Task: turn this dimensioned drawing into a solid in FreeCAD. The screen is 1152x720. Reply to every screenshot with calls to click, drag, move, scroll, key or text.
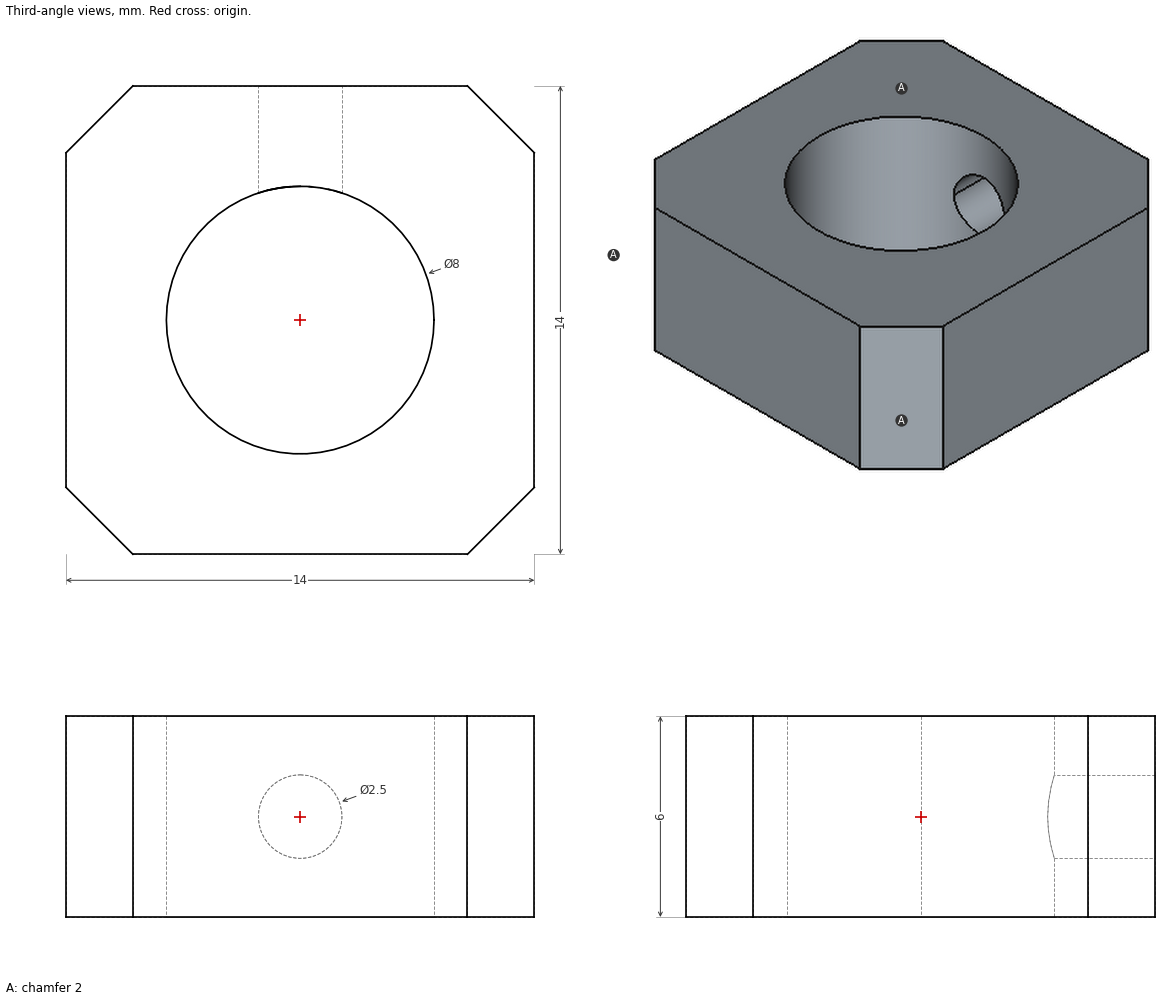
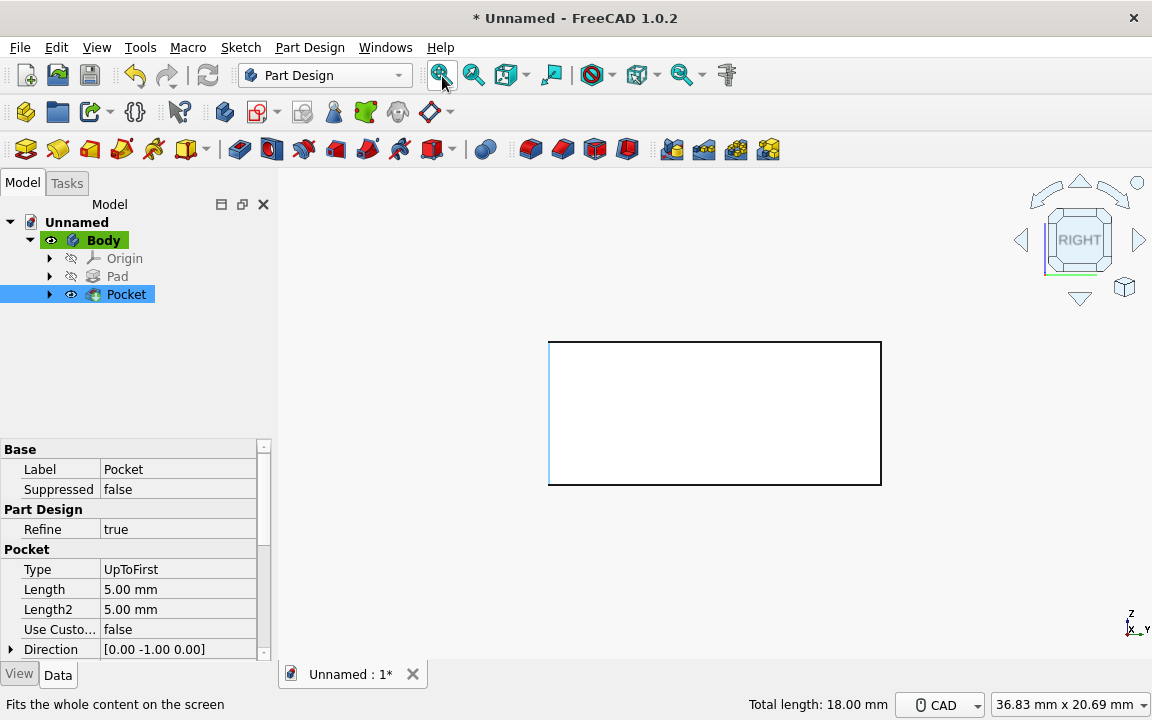
click(881, 412, ctrl)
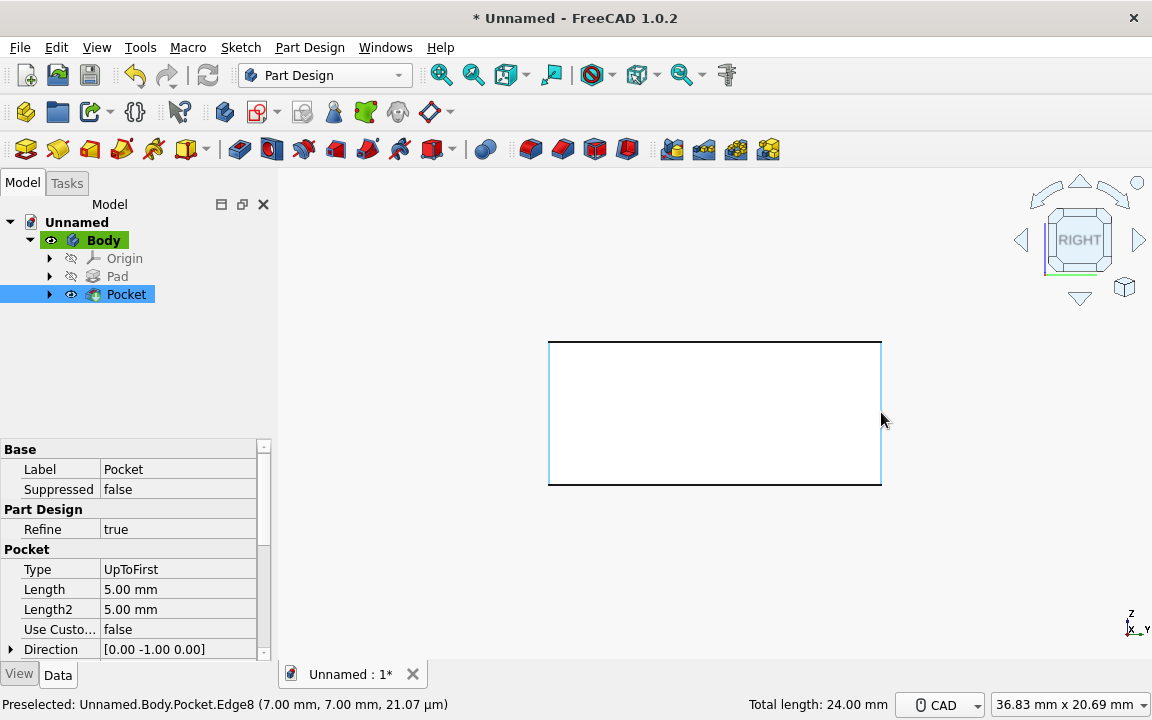
click(564, 150)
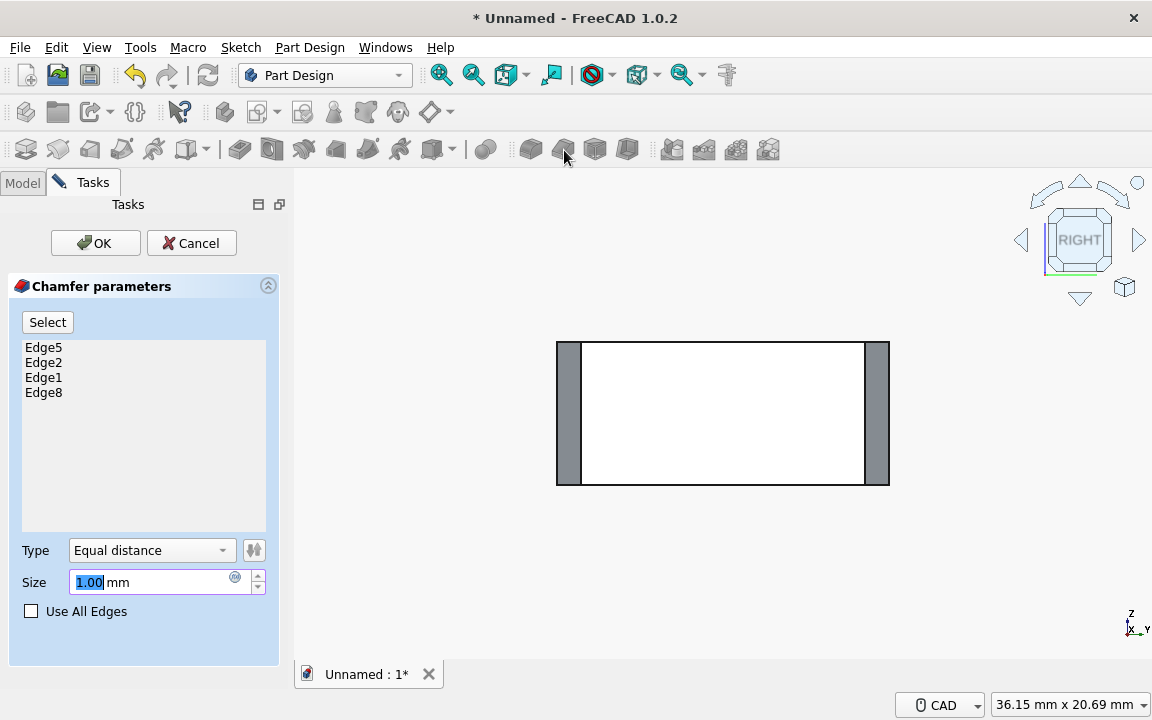
text(2)
key(Tab)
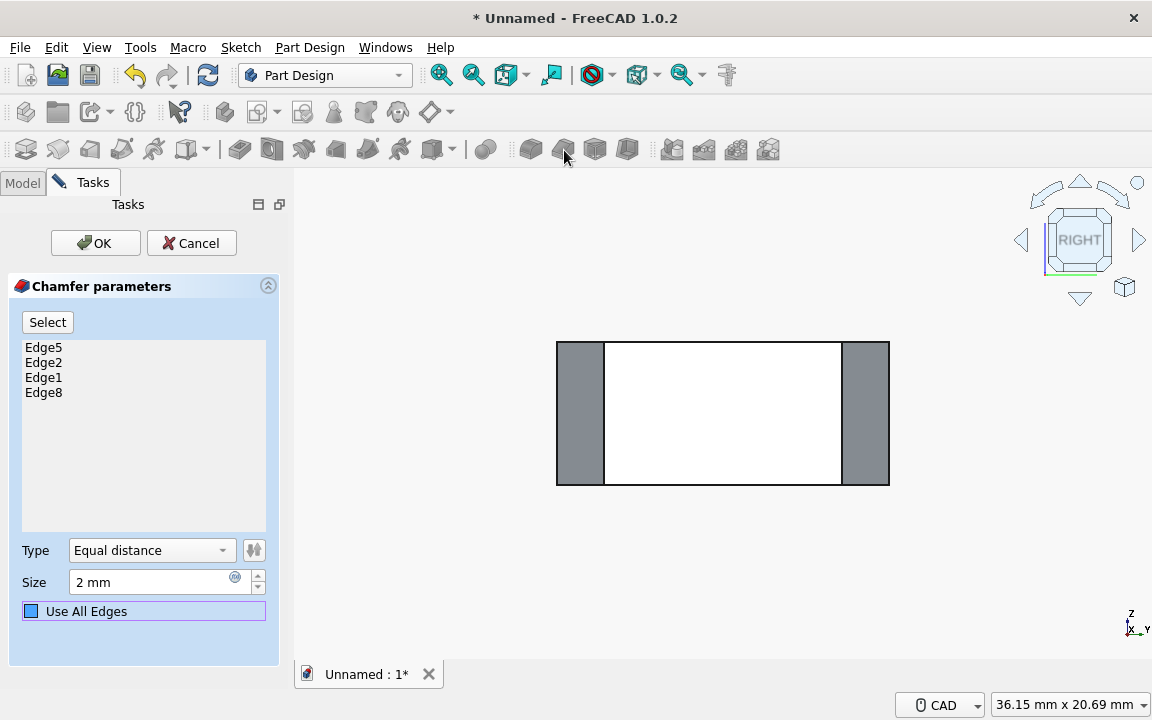
click(96, 243)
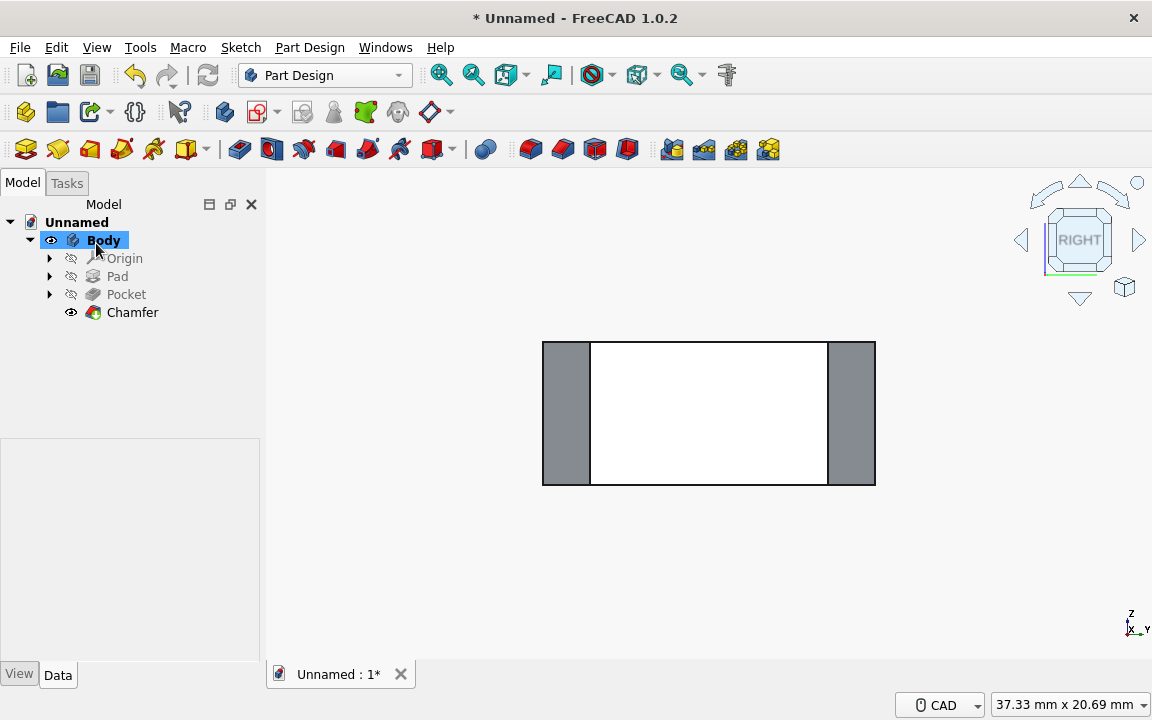
key(0)